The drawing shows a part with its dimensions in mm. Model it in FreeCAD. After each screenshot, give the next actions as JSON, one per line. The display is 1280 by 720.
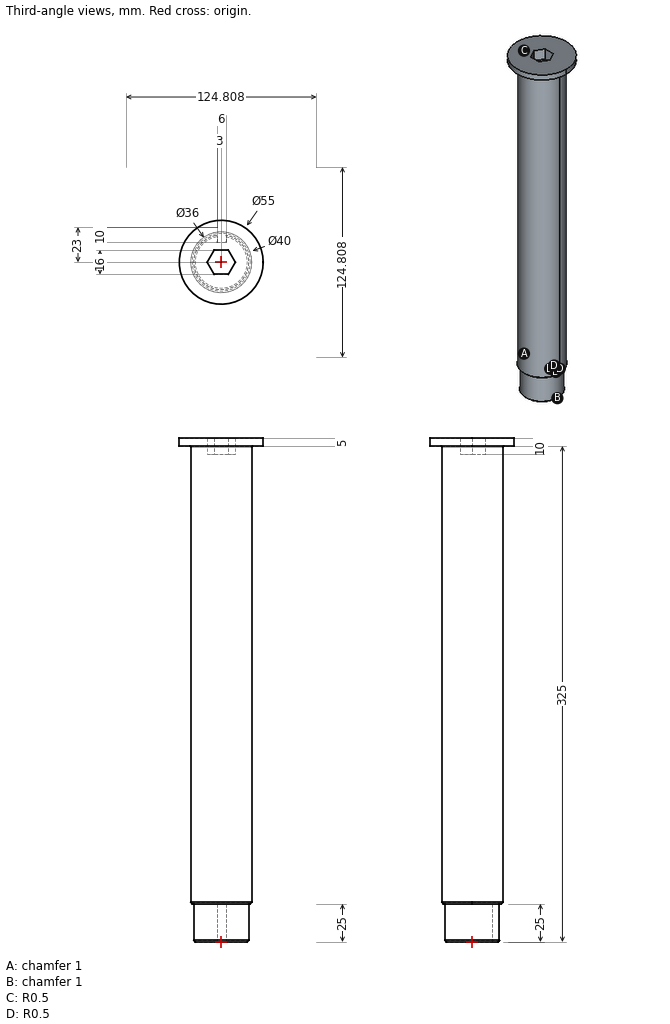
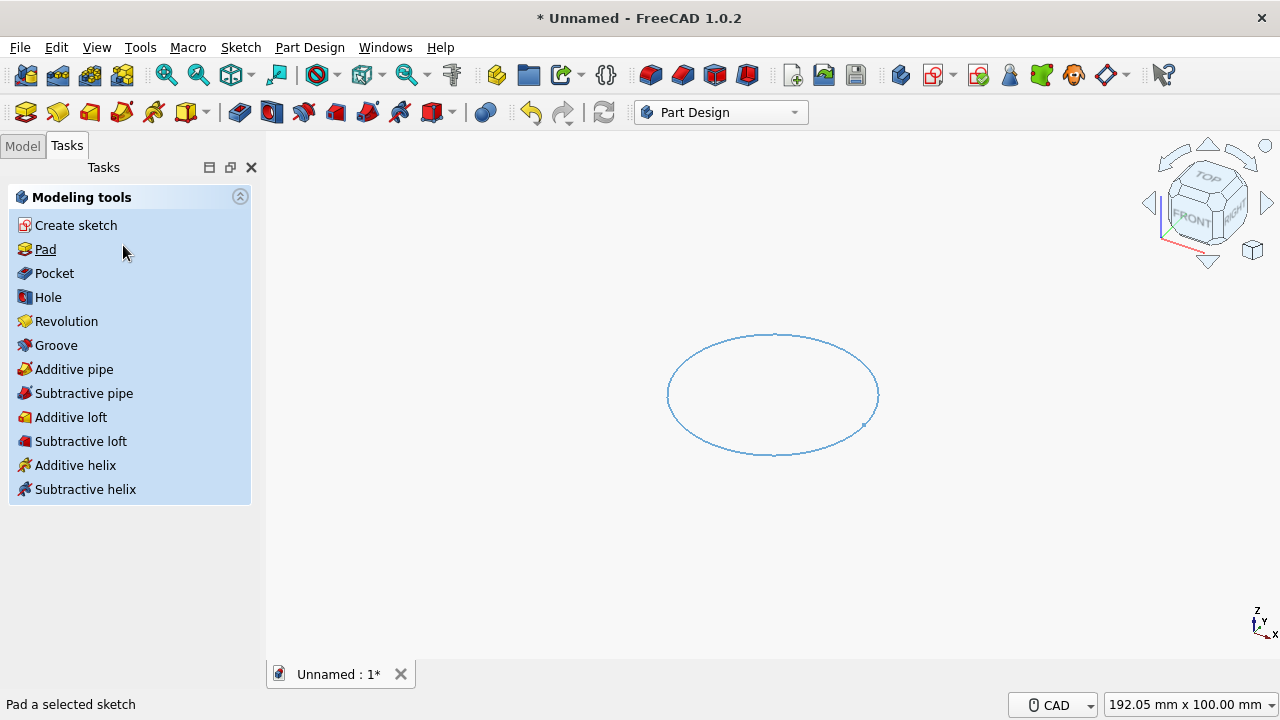
{"action": "left_click", "coordinate": [26, 112]}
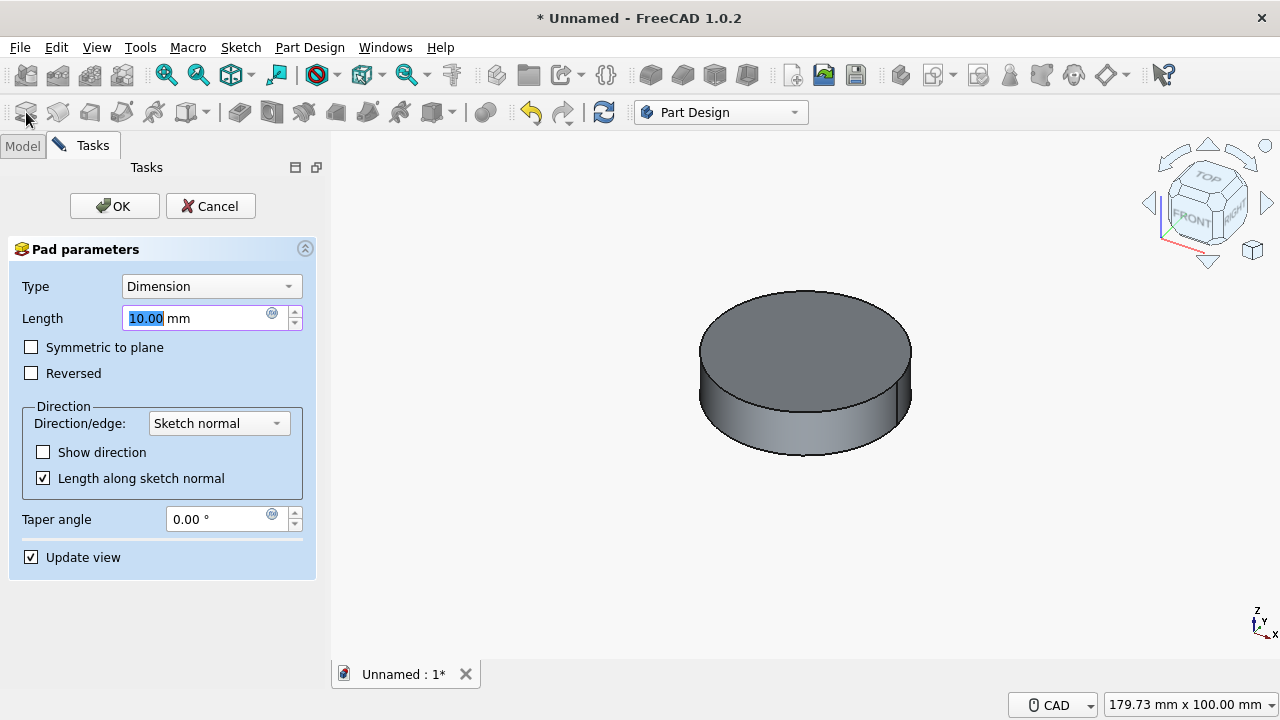
{"action": "type", "text": "325"}
{"action": "key", "text": "Tab"}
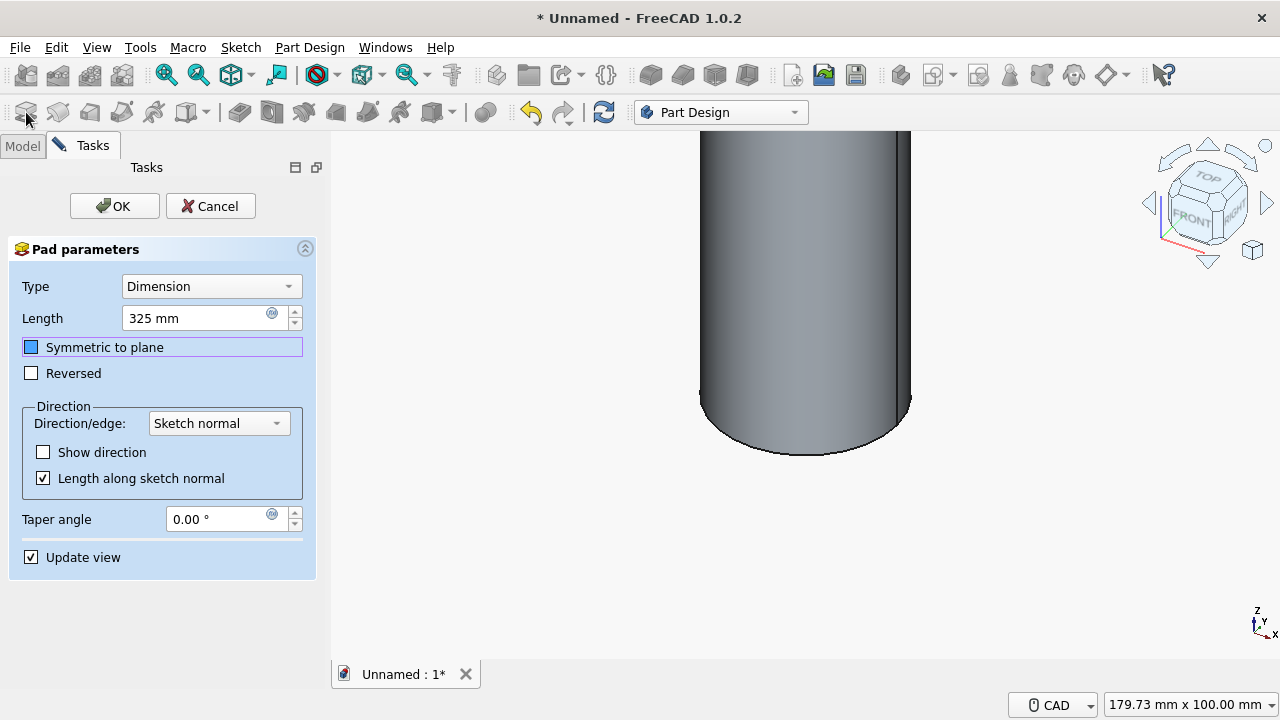
{"action": "left_click", "coordinate": [115, 206]}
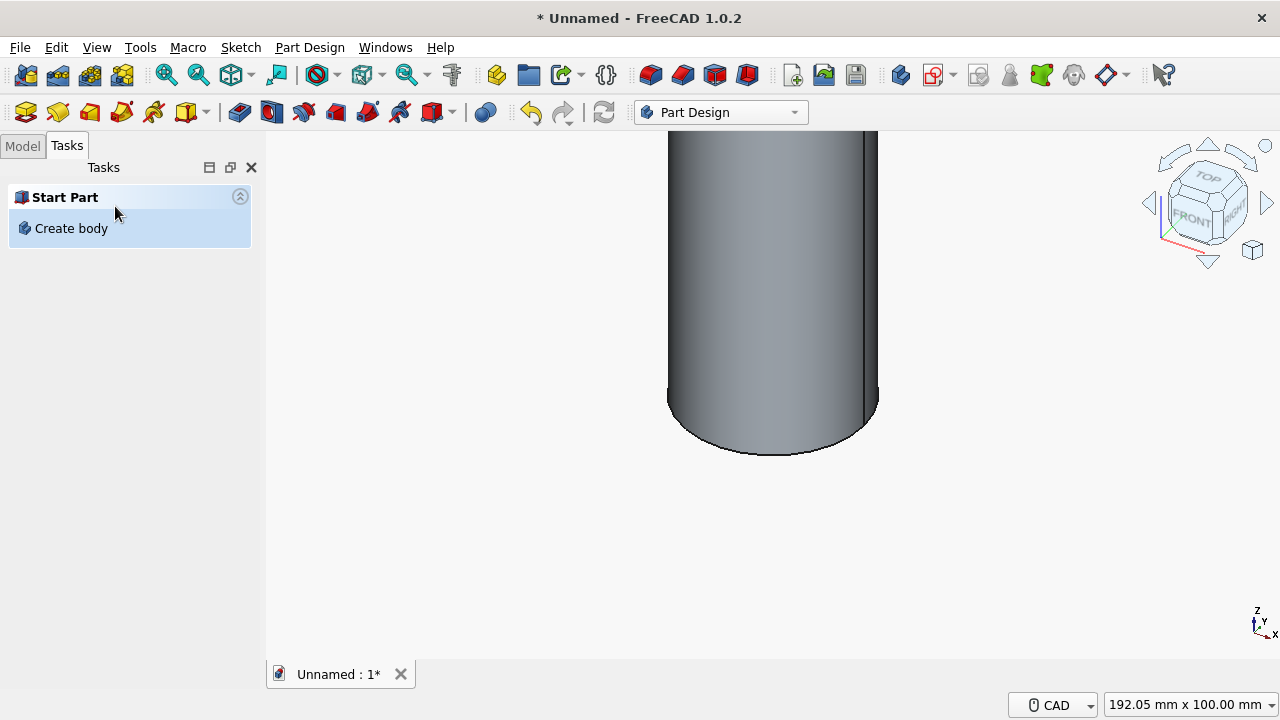
{"action": "left_click", "coordinate": [168, 76]}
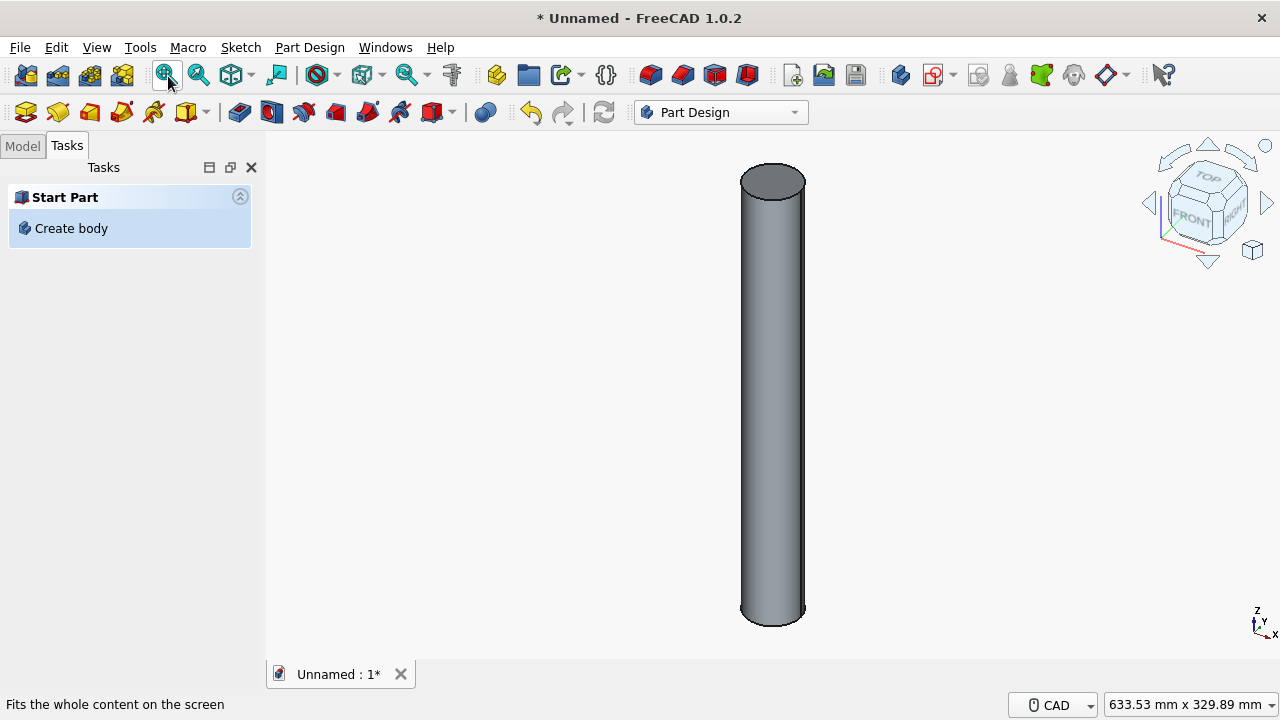
{"action": "left_click", "coordinate": [773, 181]}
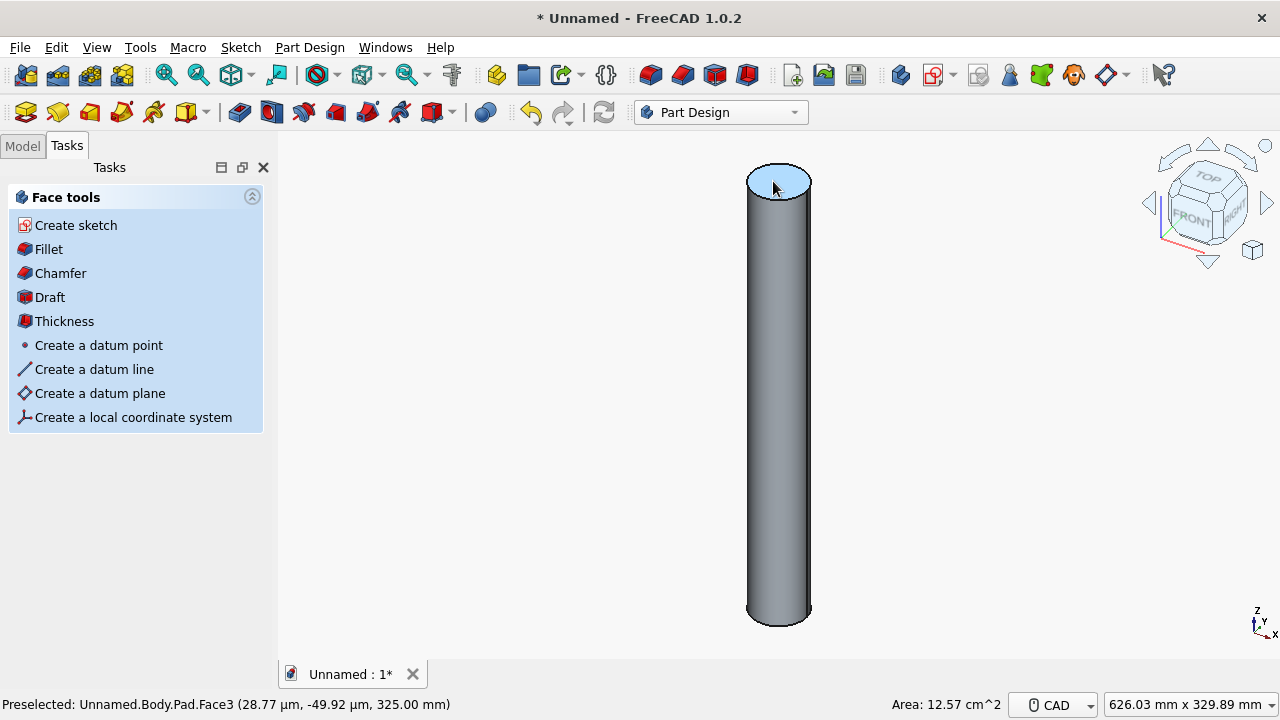
{"action": "left_click", "coordinate": [934, 76]}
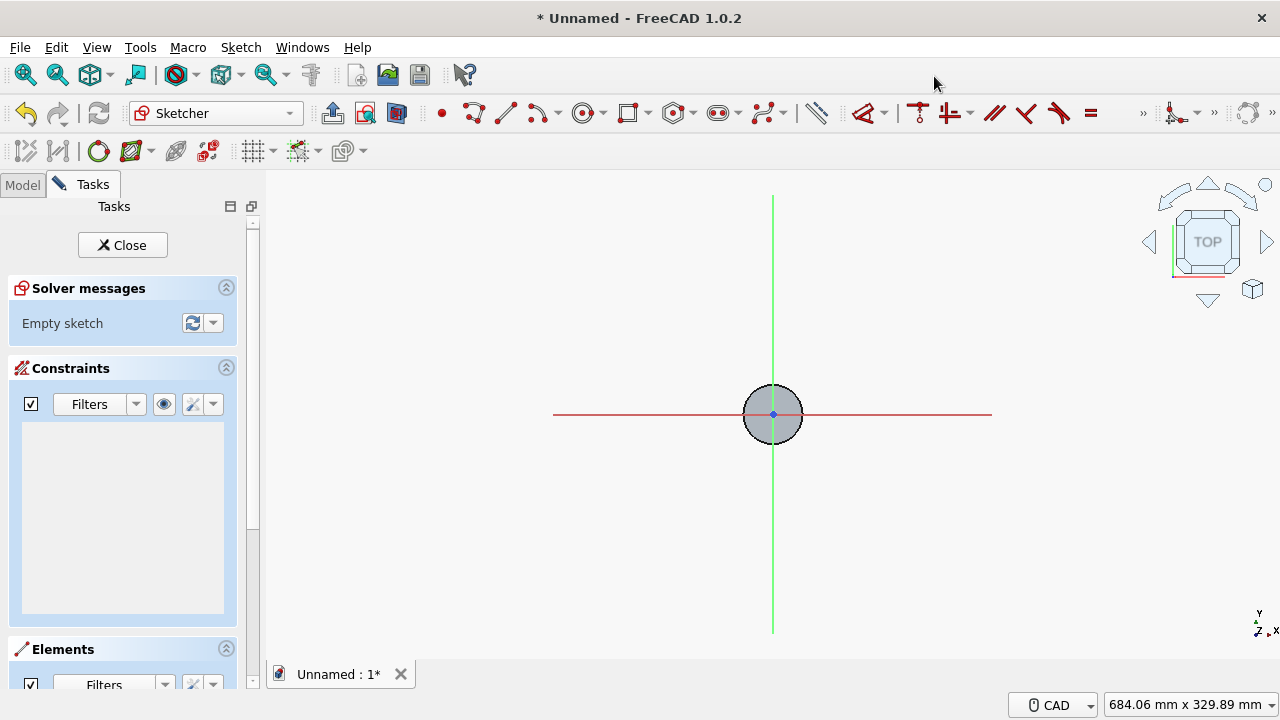
{"action": "scroll", "coordinate": [795, 415], "scroll_direction": "up", "scroll_amount": 7}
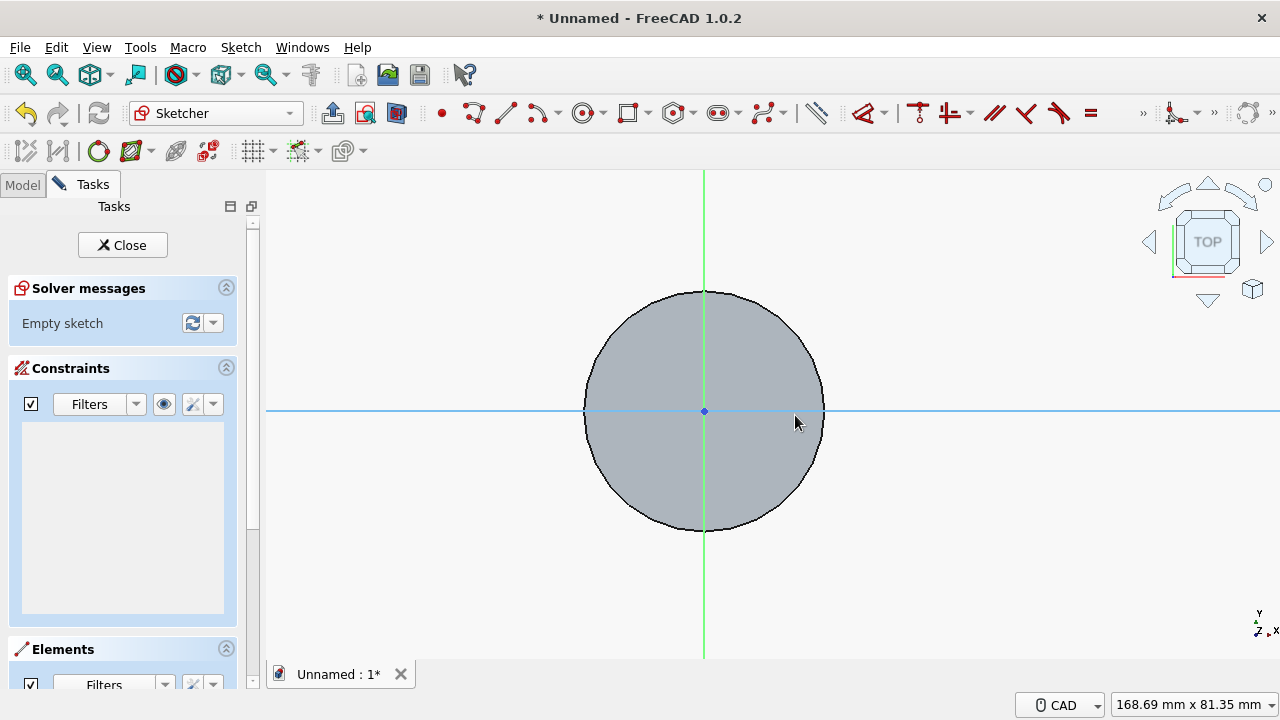
{"action": "left_click", "coordinate": [584, 114]}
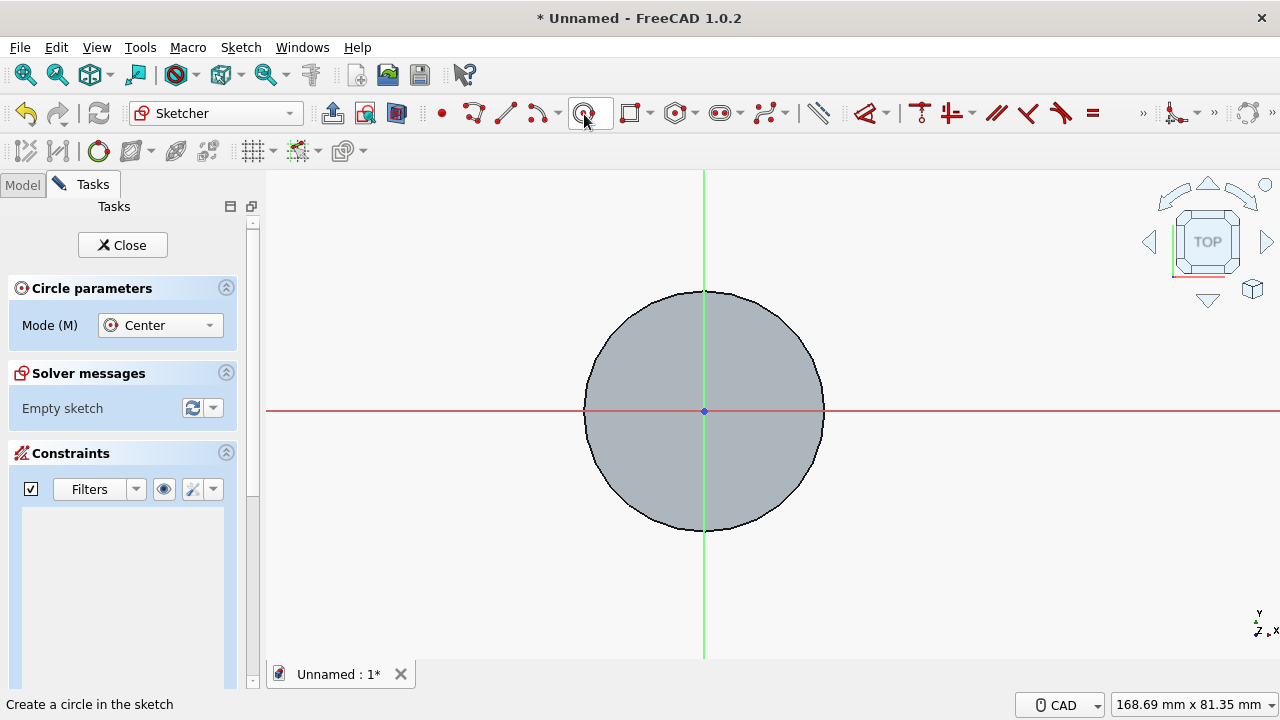
{"action": "left_click", "coordinate": [704, 411]}
{"action": "left_click", "coordinate": [821, 295]}
{"action": "key", "text": "Escape"}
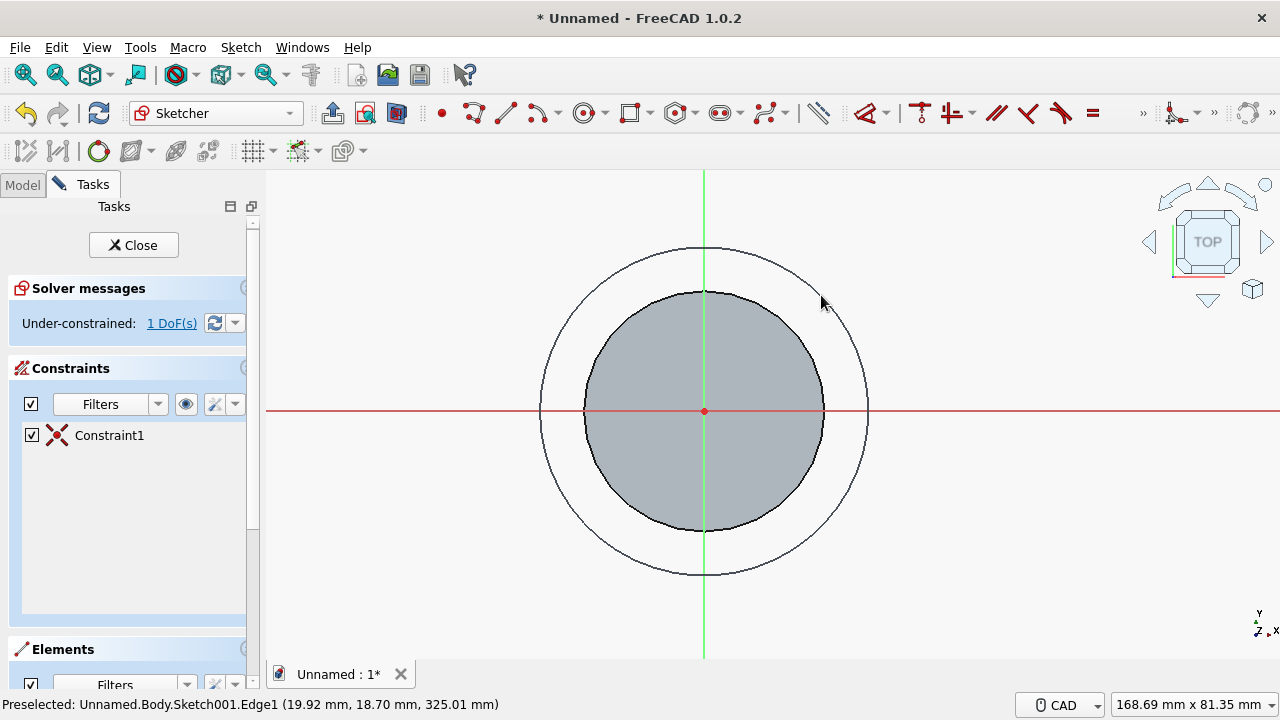
{"action": "left_click", "coordinate": [866, 114]}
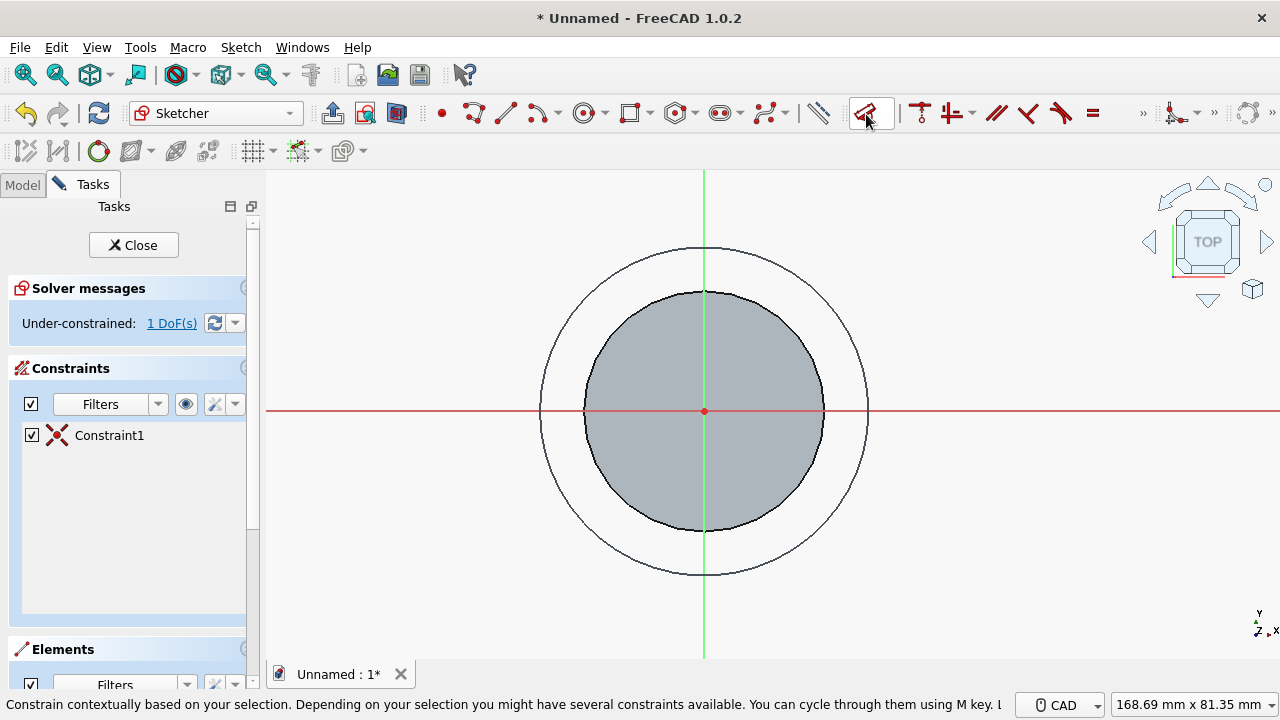
{"action": "left_click", "coordinate": [820, 295]}
{"action": "left_click", "coordinate": [843, 272]}